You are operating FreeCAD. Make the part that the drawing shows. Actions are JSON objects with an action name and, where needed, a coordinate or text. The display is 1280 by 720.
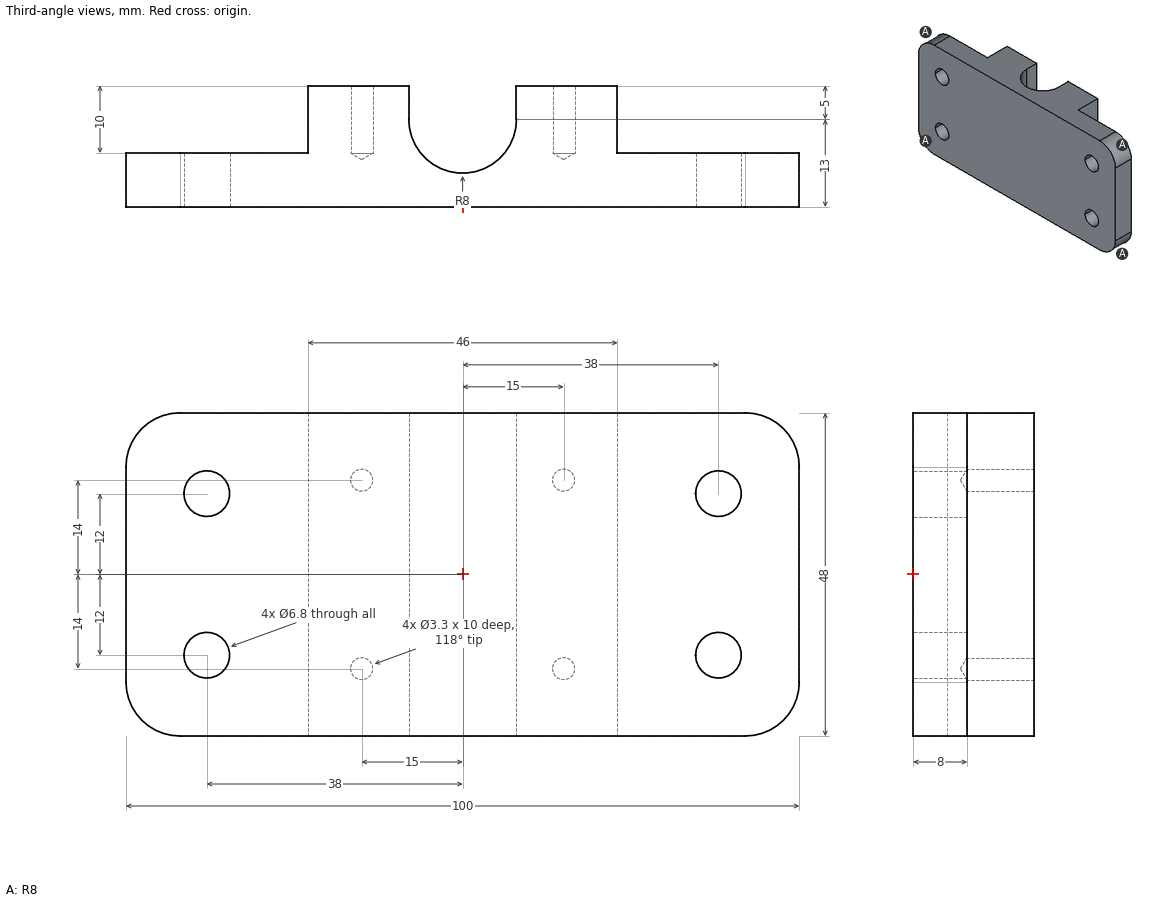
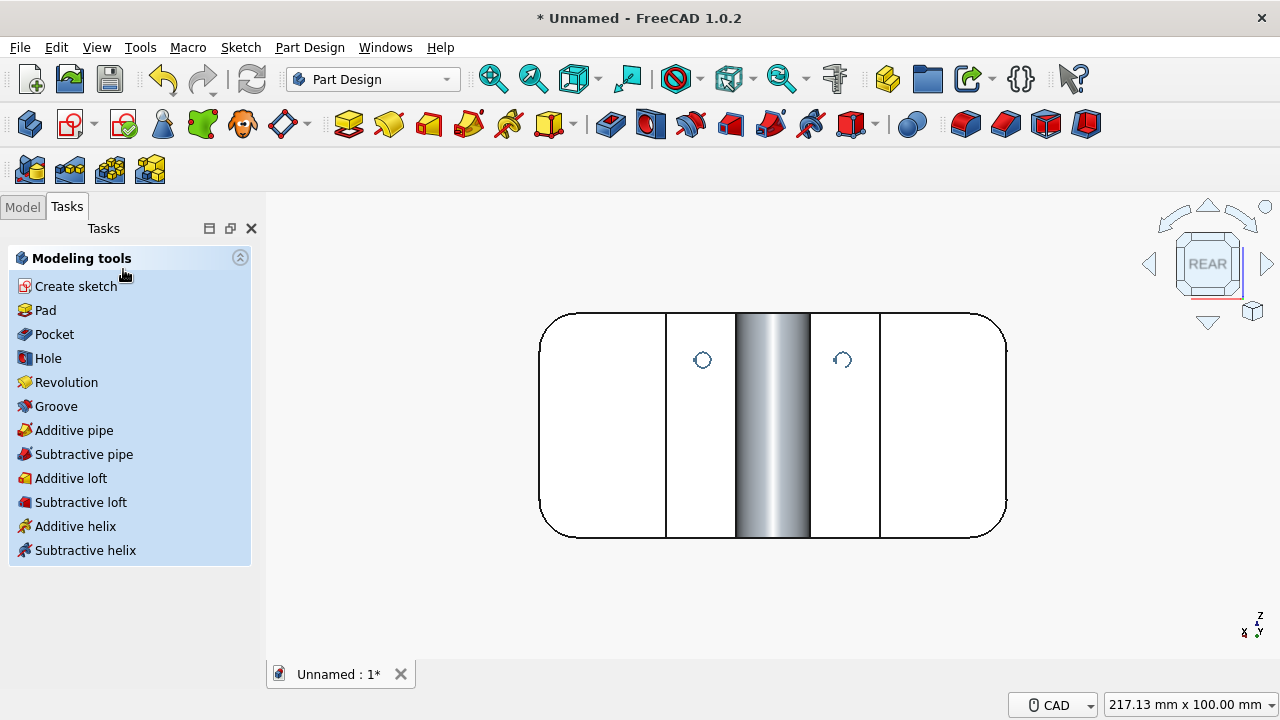
{"action": "left_click", "coordinate": [652, 124]}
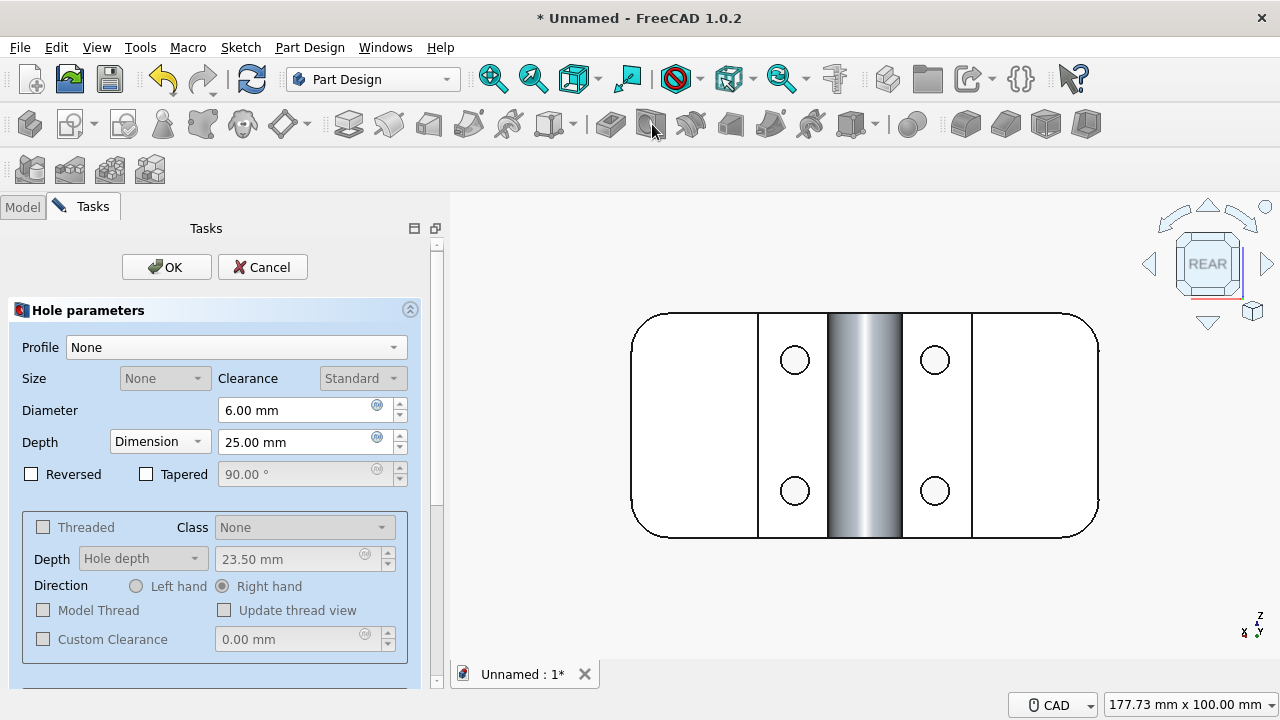
{"action": "triple_click", "coordinate": [305, 410]}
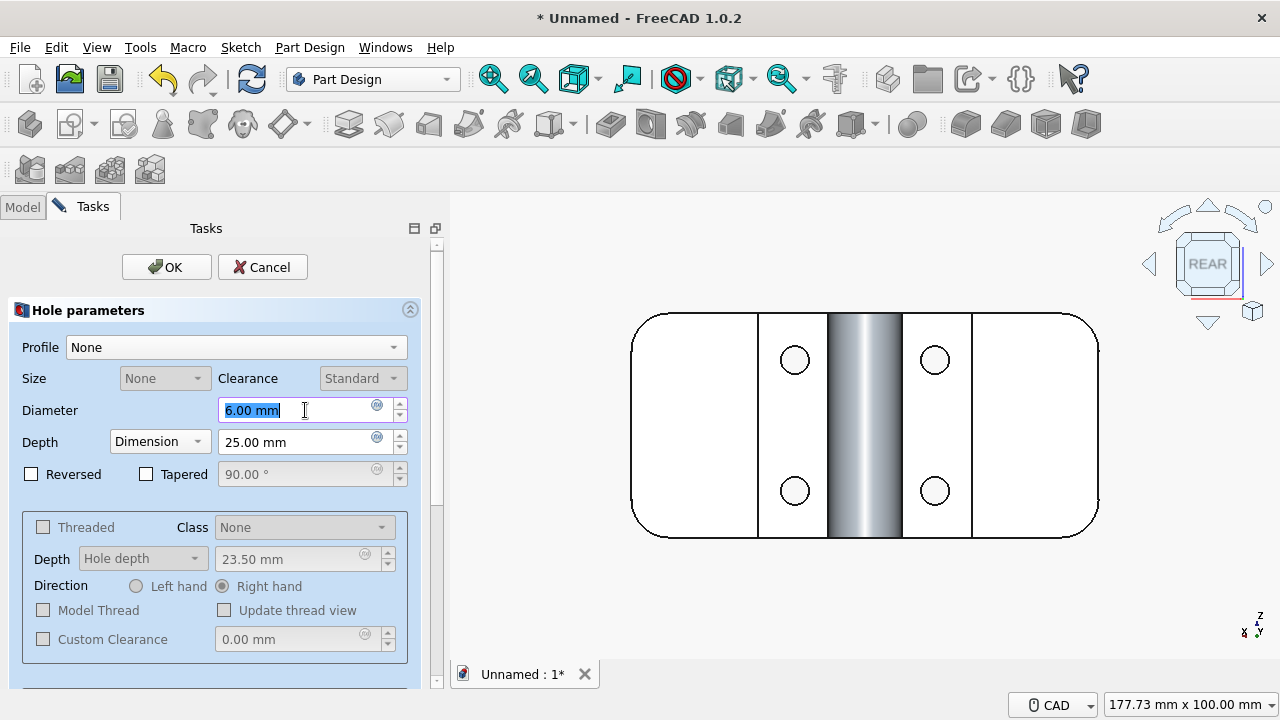
{"action": "type", "text": "3.3"}
{"action": "key", "text": "Tab"}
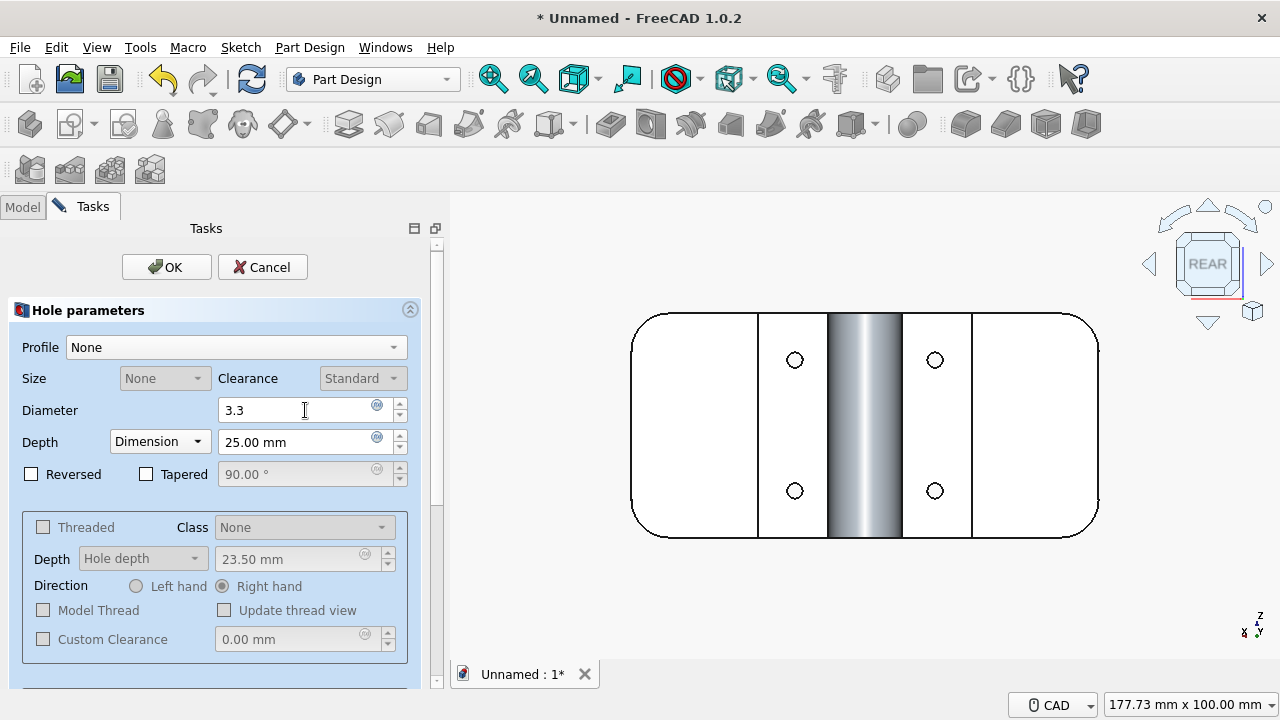
{"action": "triple_click", "coordinate": [305, 442]}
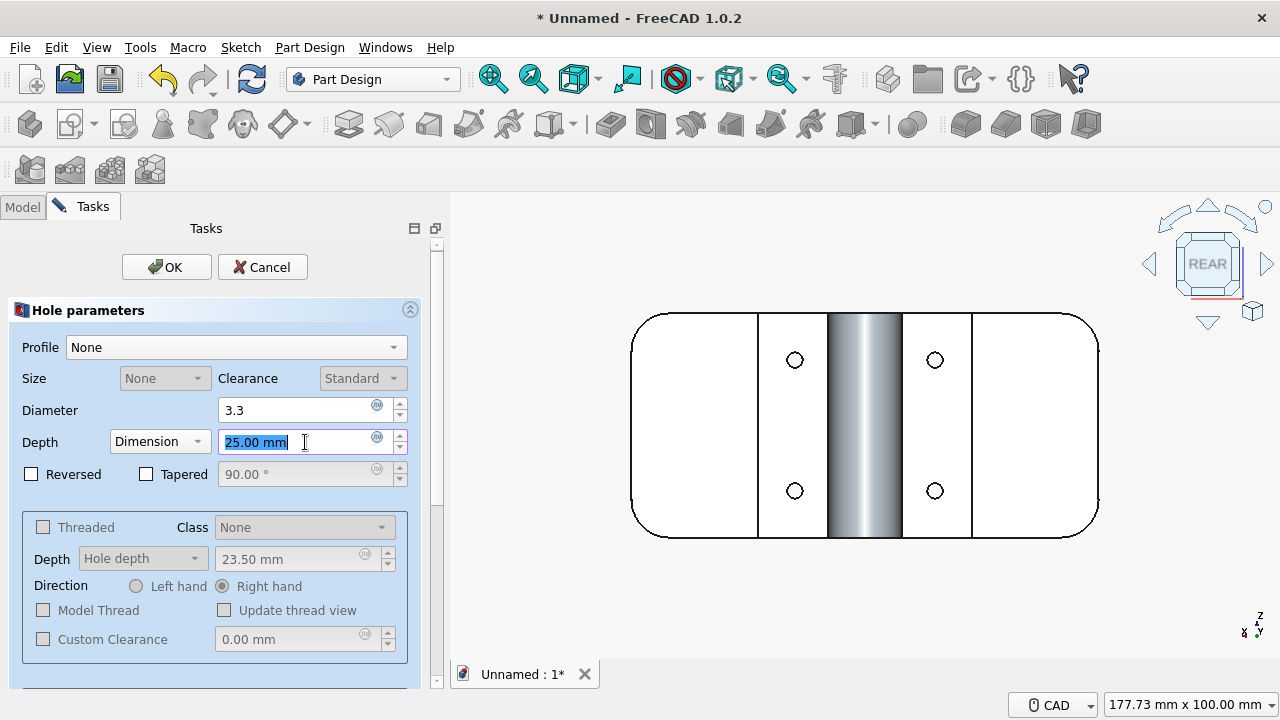
{"action": "type", "text": "10"}
{"action": "key", "text": "Tab"}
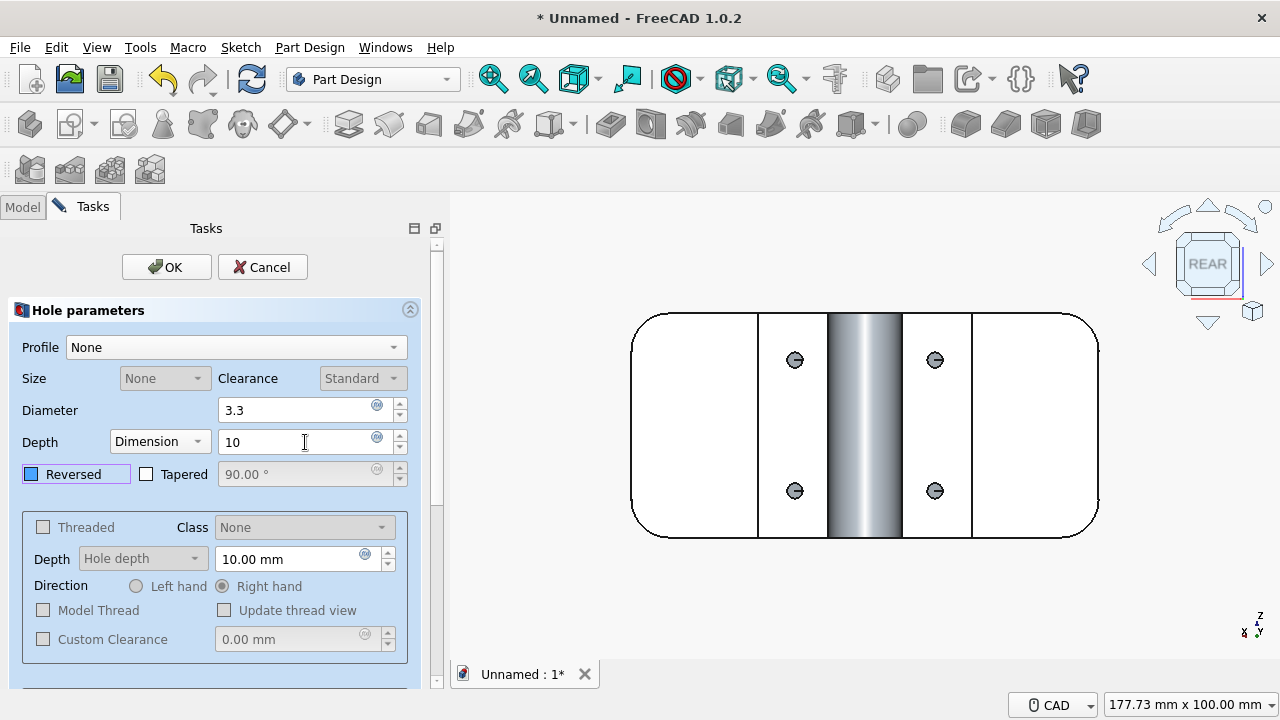
{"action": "left_click", "coordinate": [167, 267]}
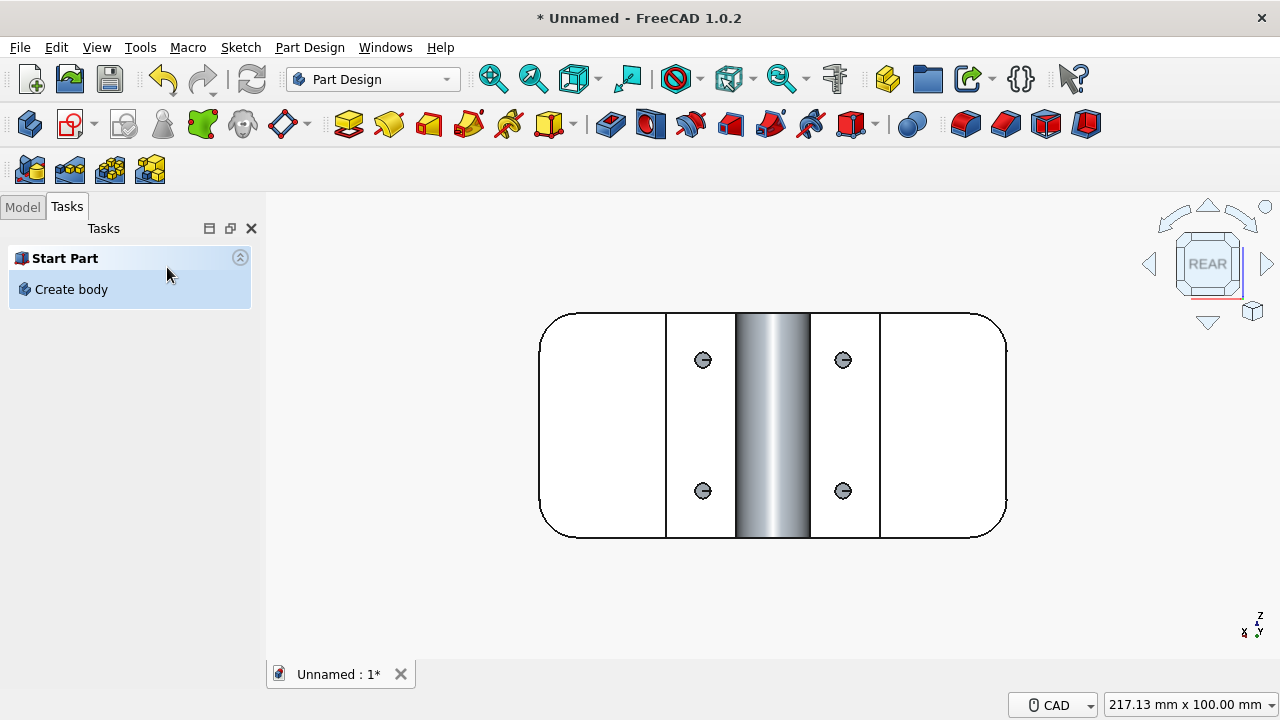
{"action": "left_click", "coordinate": [603, 392]}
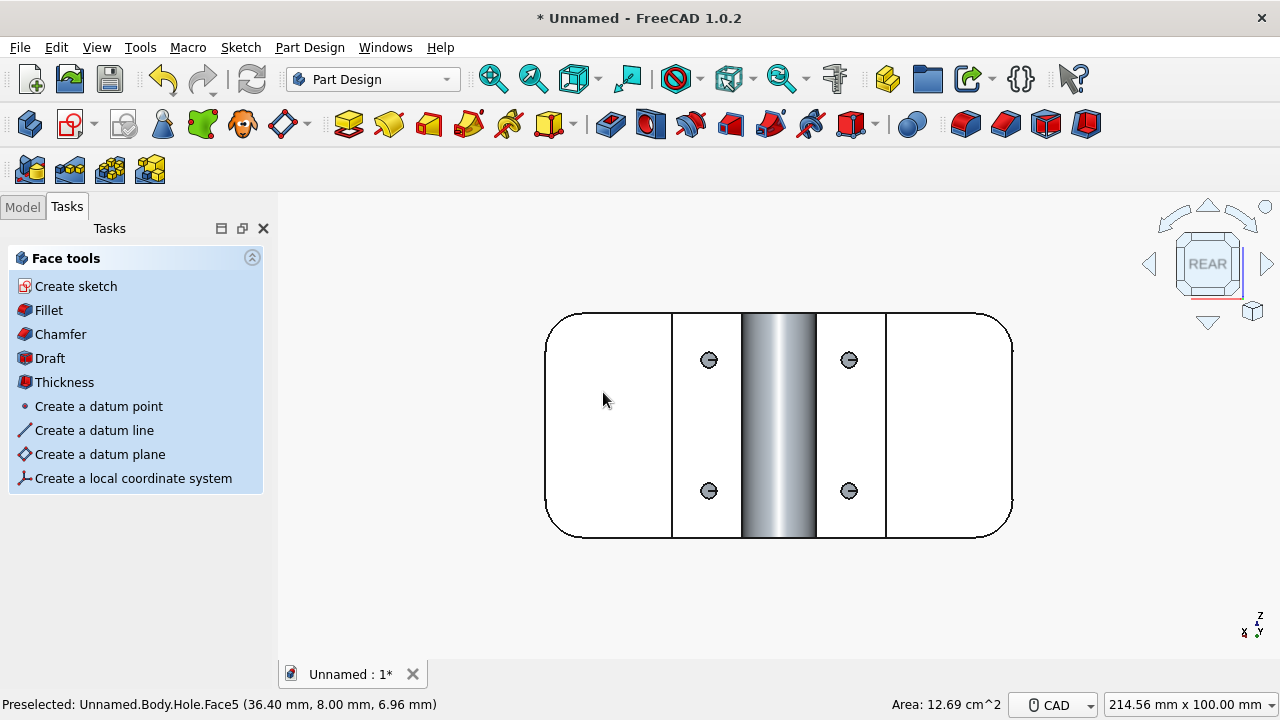
{"action": "left_click", "coordinate": [70, 124]}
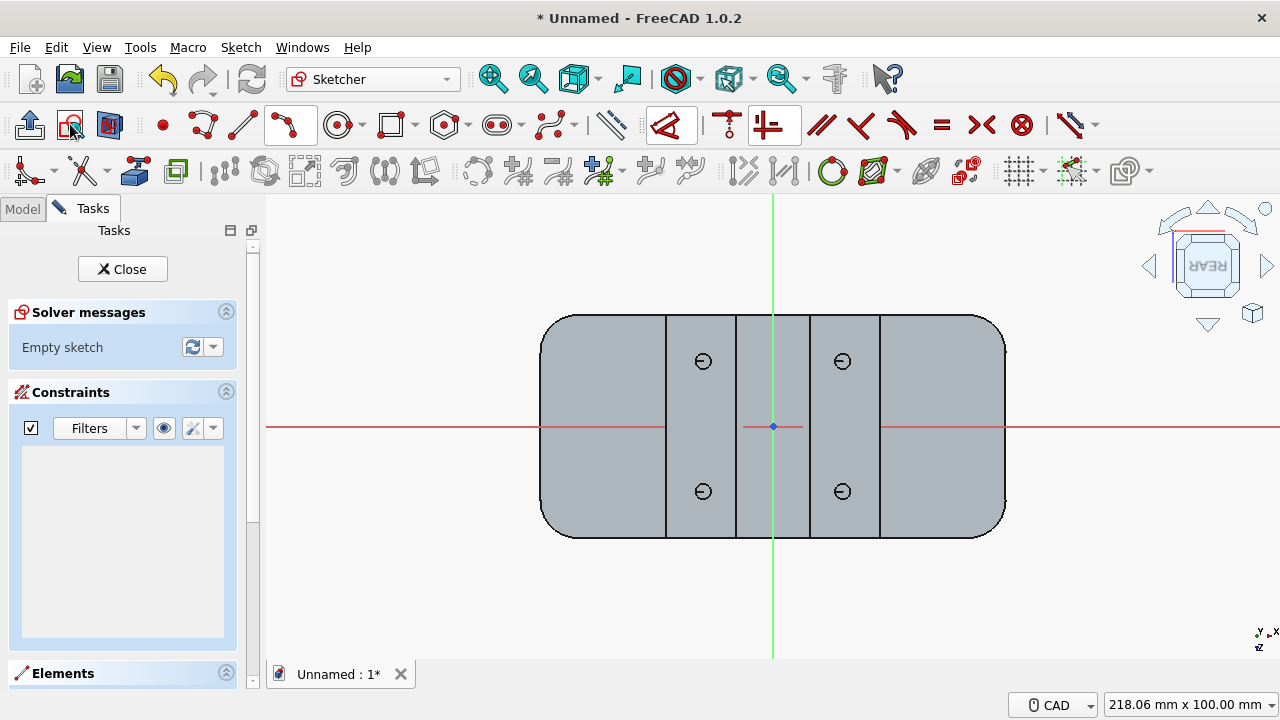
{"action": "left_click", "coordinate": [110, 126]}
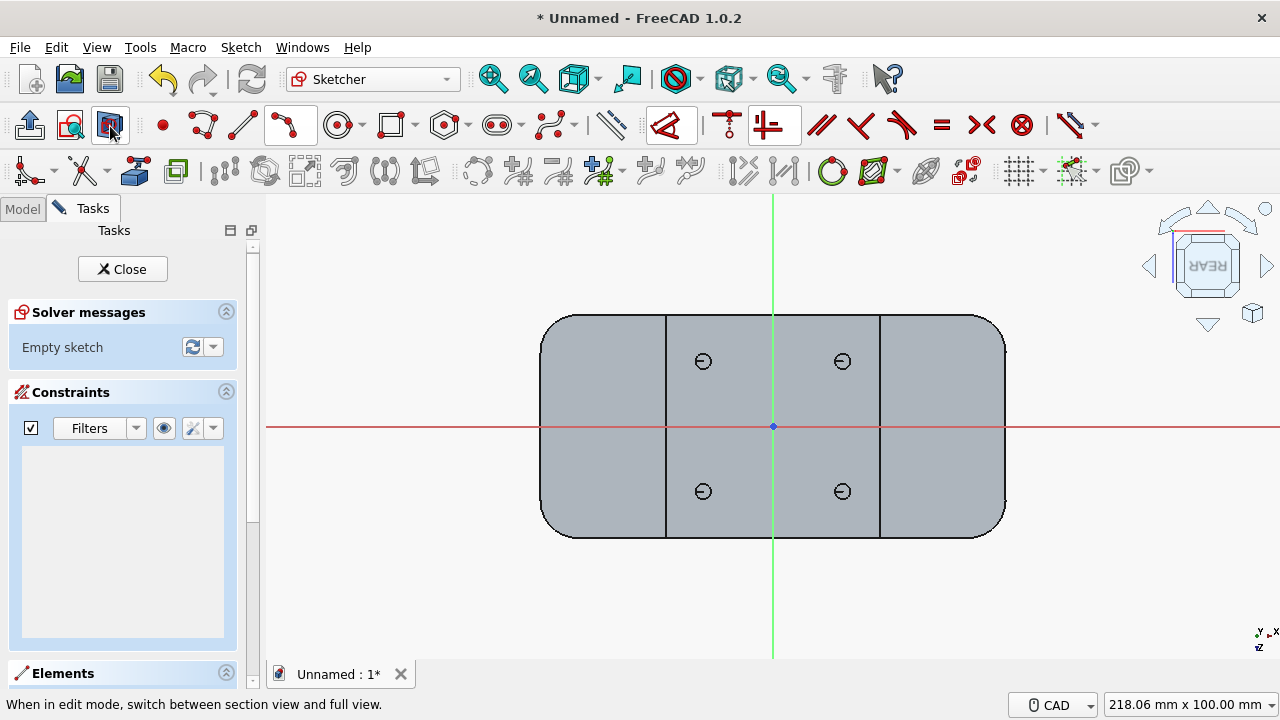
{"action": "scroll", "coordinate": [912, 426], "scroll_direction": "up", "scroll_amount": 2}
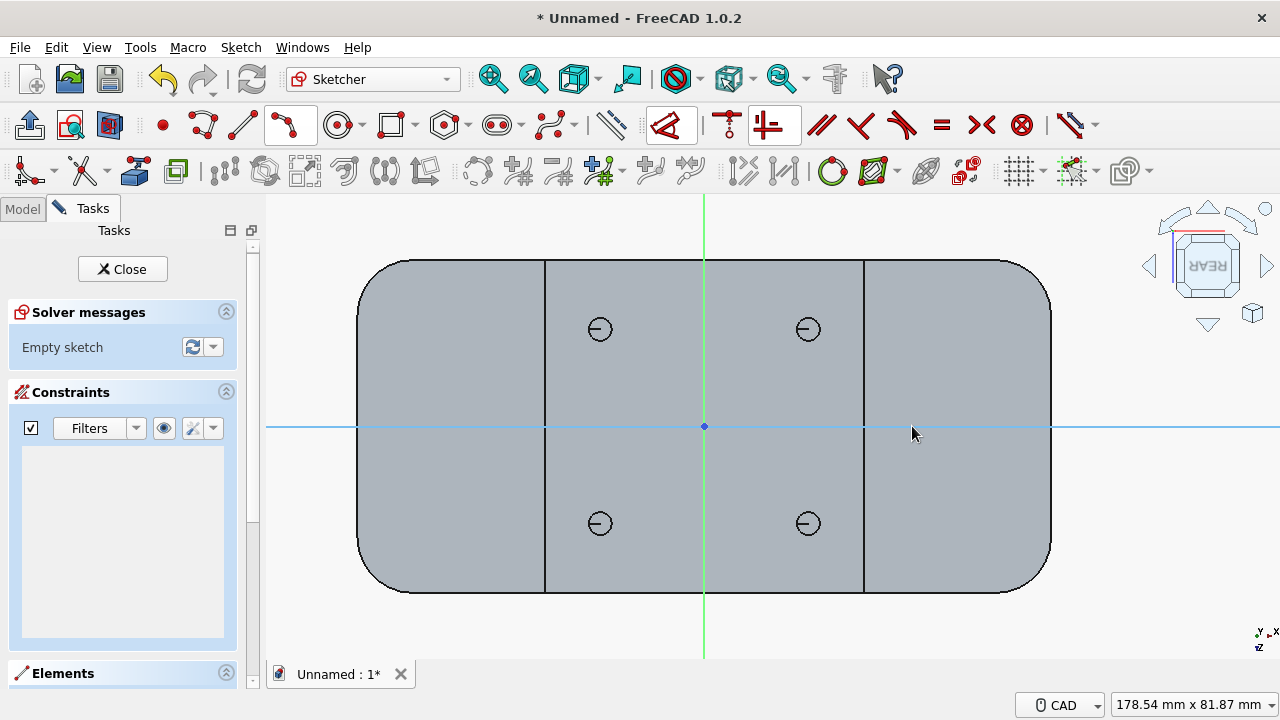
{"action": "key", "text": "g c"}